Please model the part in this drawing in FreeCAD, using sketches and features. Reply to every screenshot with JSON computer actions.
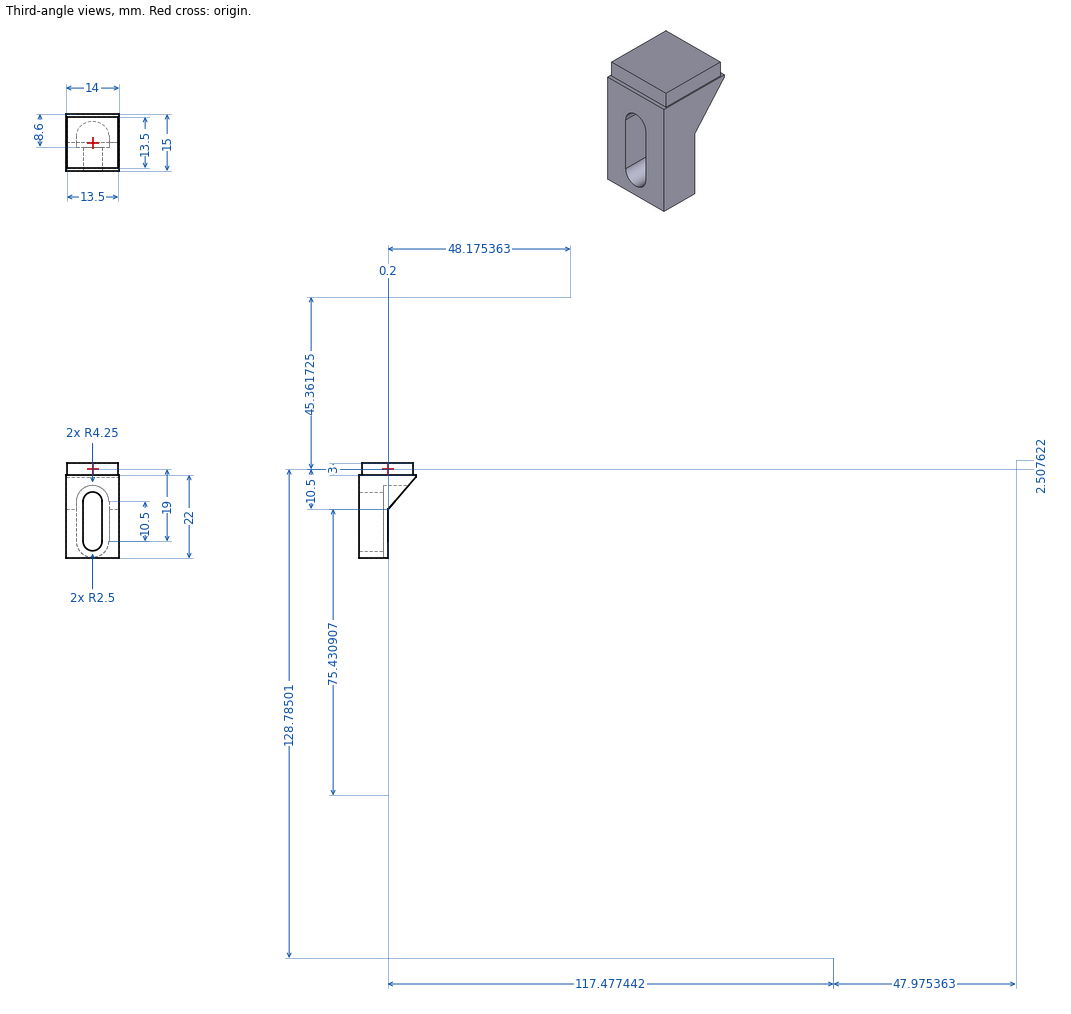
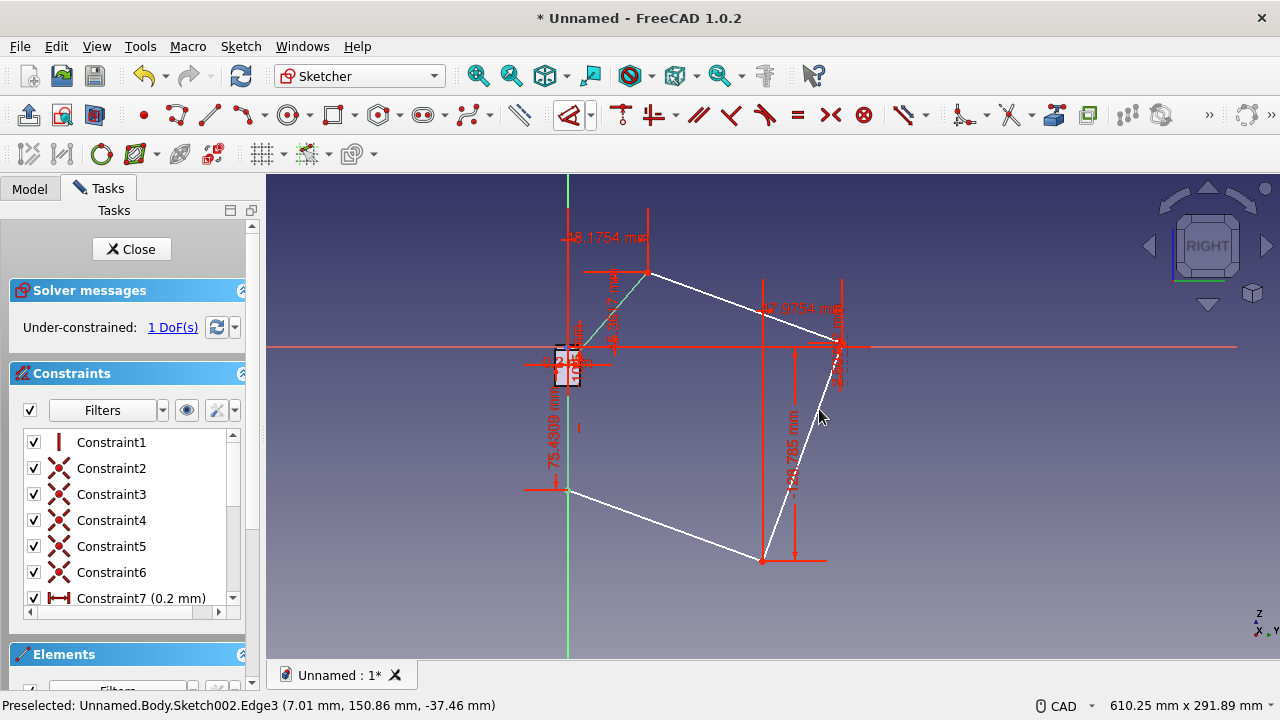
{"action": "left_click", "coordinate": [763, 561]}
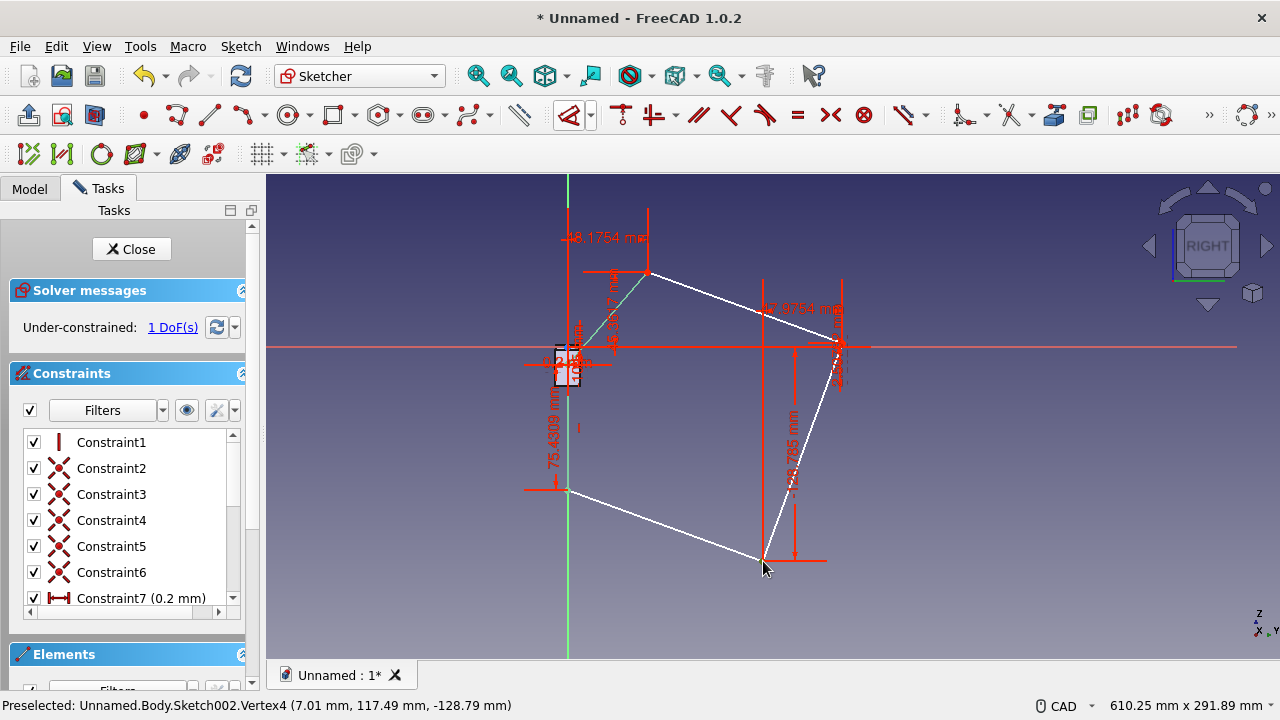
{"action": "key", "text": "l"}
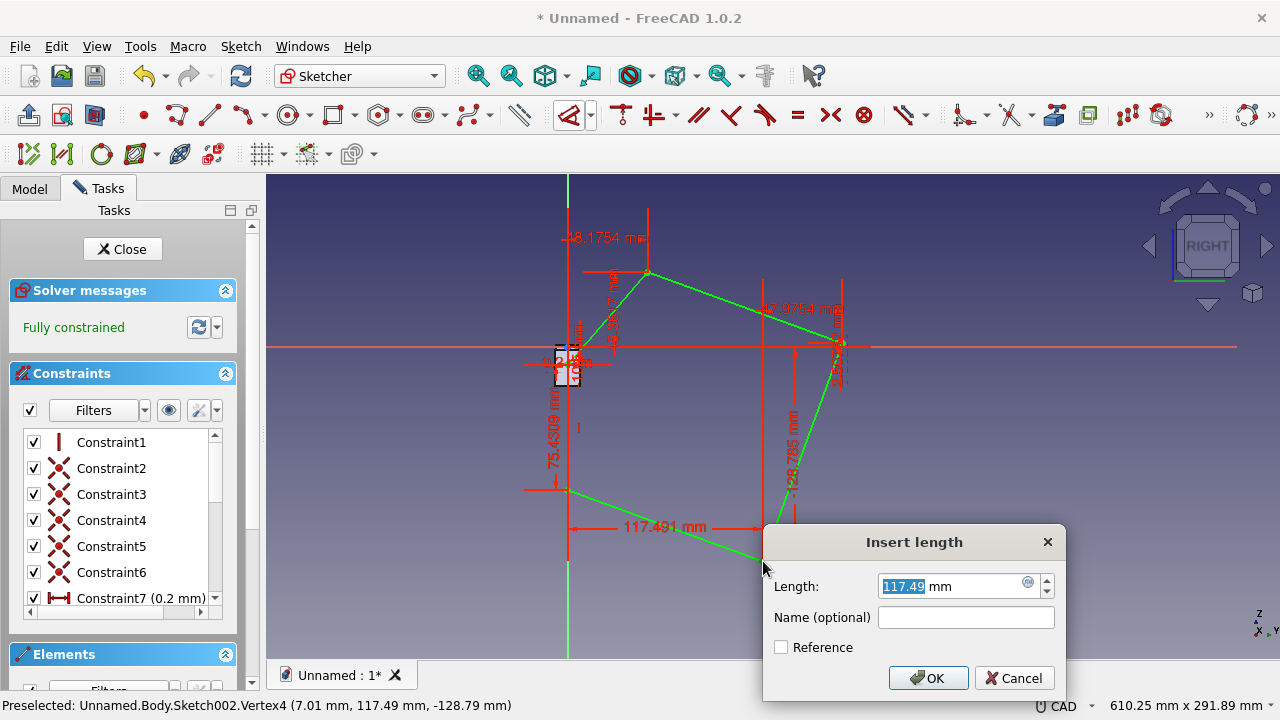
{"action": "type", "text": "117.477442"}
{"action": "key", "text": "Return"}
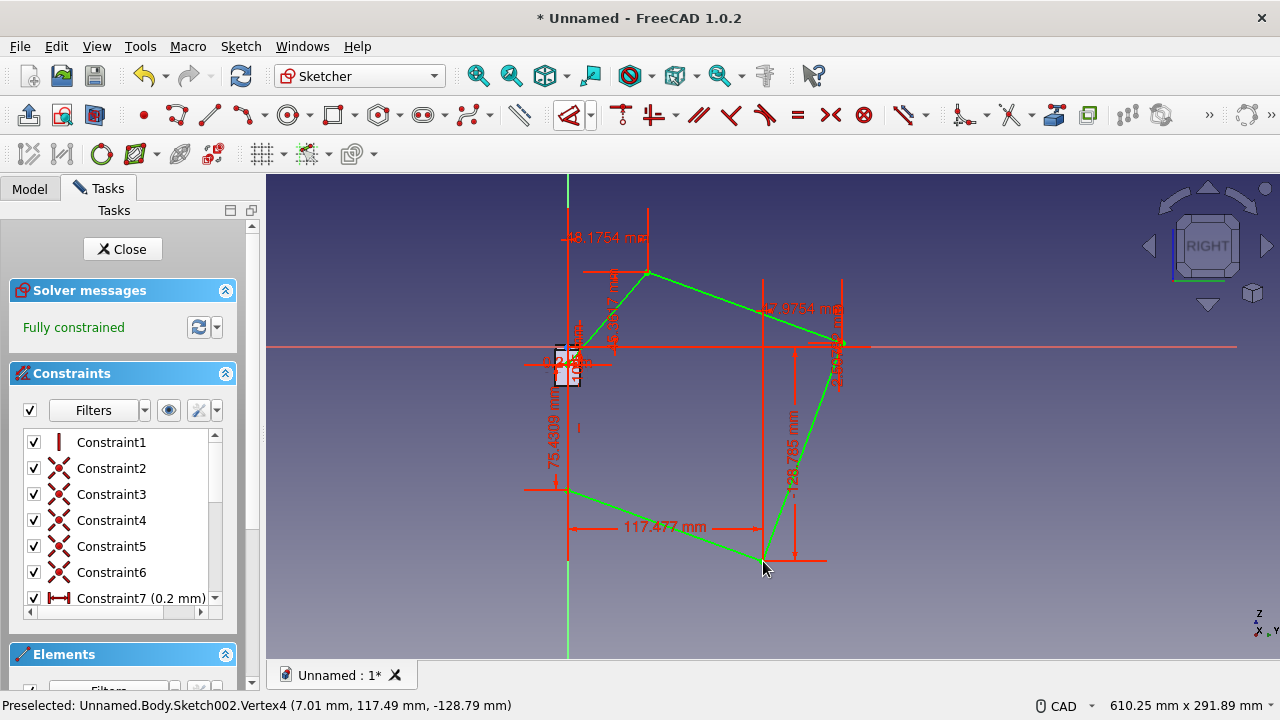
{"action": "left_click", "coordinate": [123, 249]}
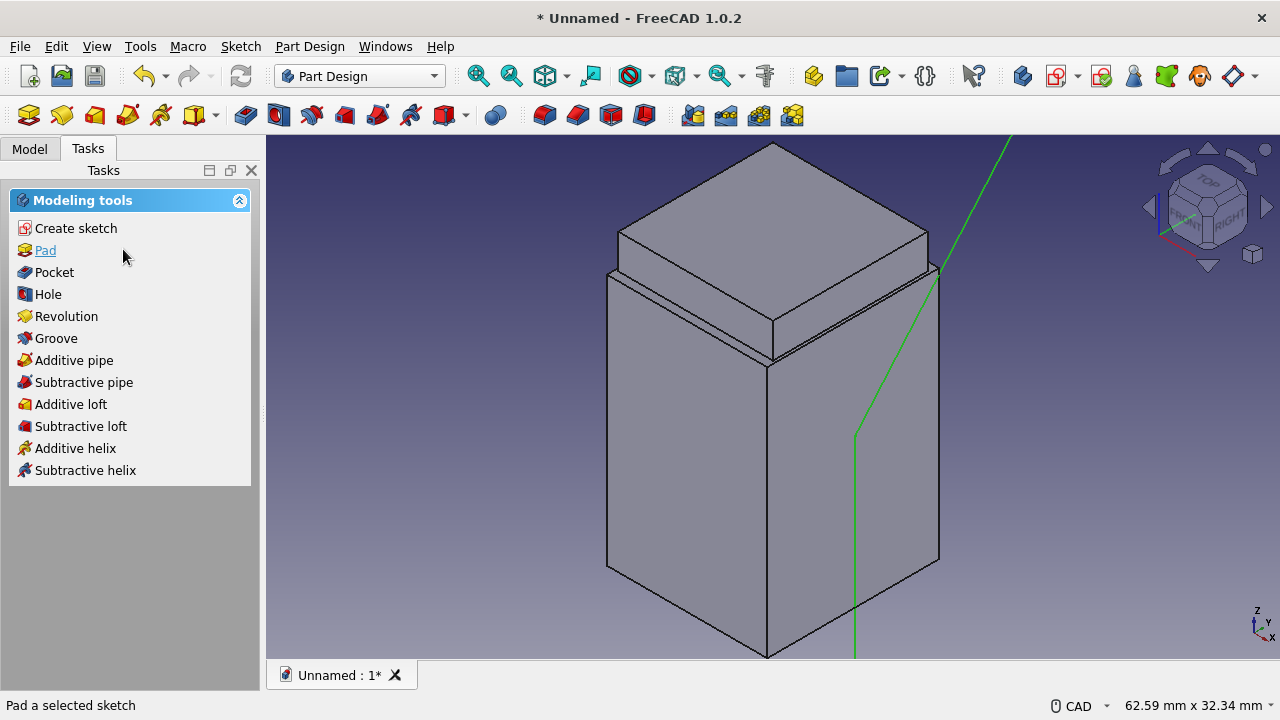
{"action": "left_click", "coordinate": [246, 116]}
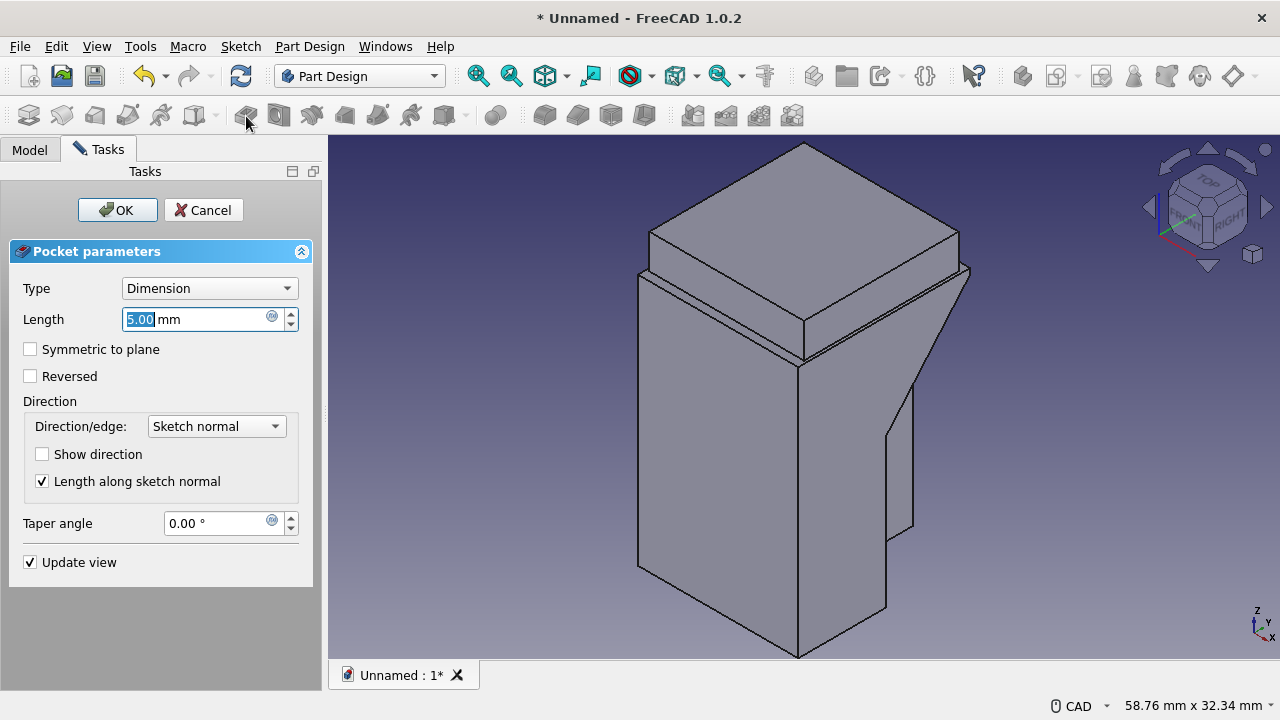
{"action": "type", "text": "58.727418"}
{"action": "key", "text": "Tab"}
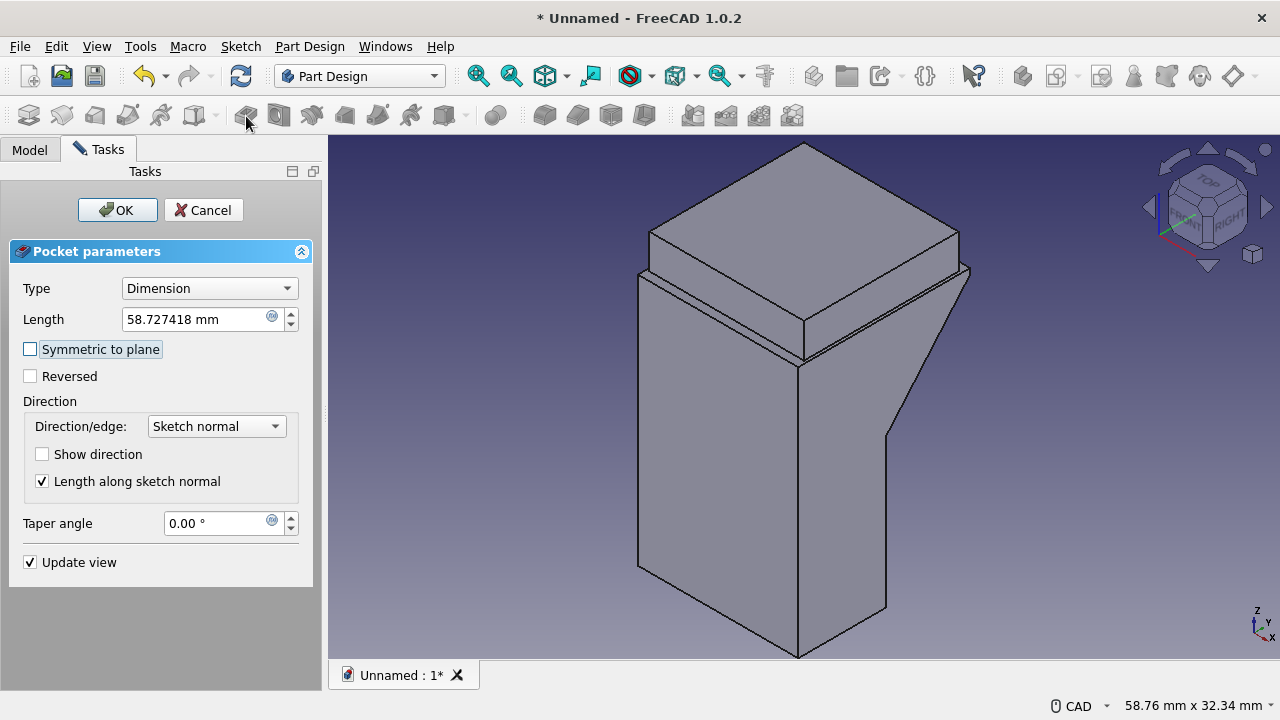
{"action": "left_click", "coordinate": [31, 349]}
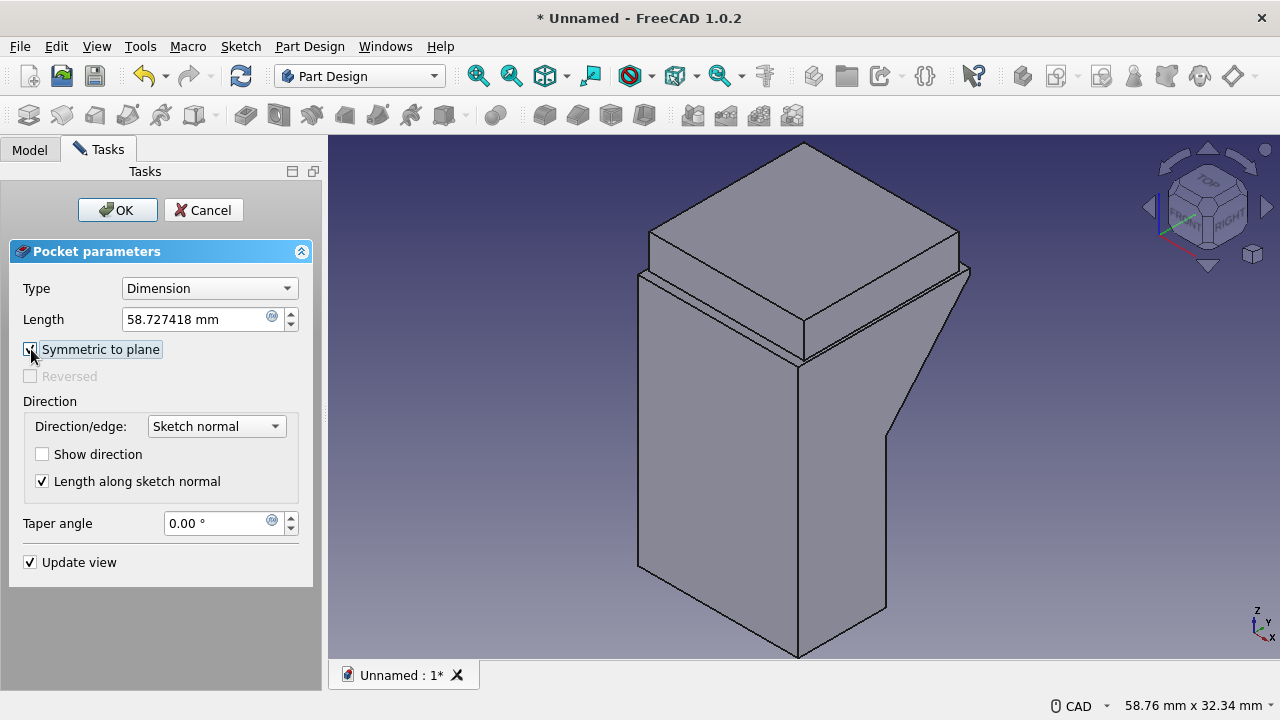
{"action": "left_click", "coordinate": [118, 210]}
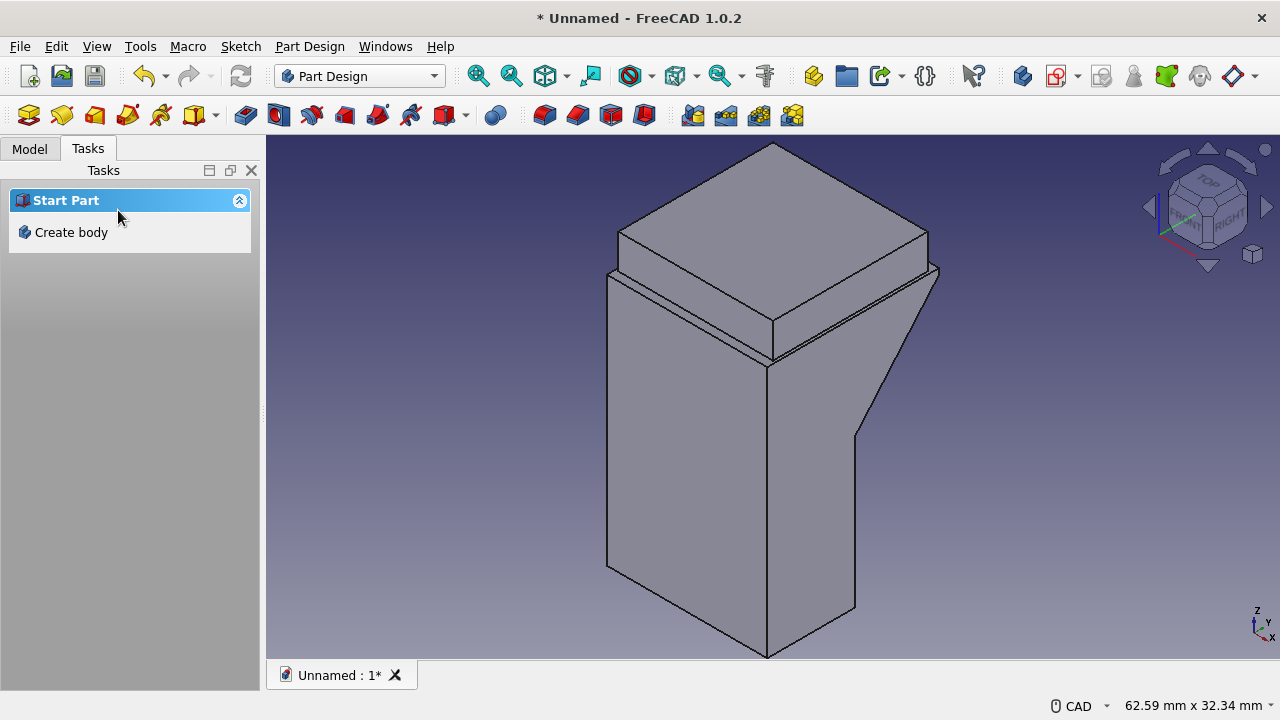
{"action": "key", "text": "4"}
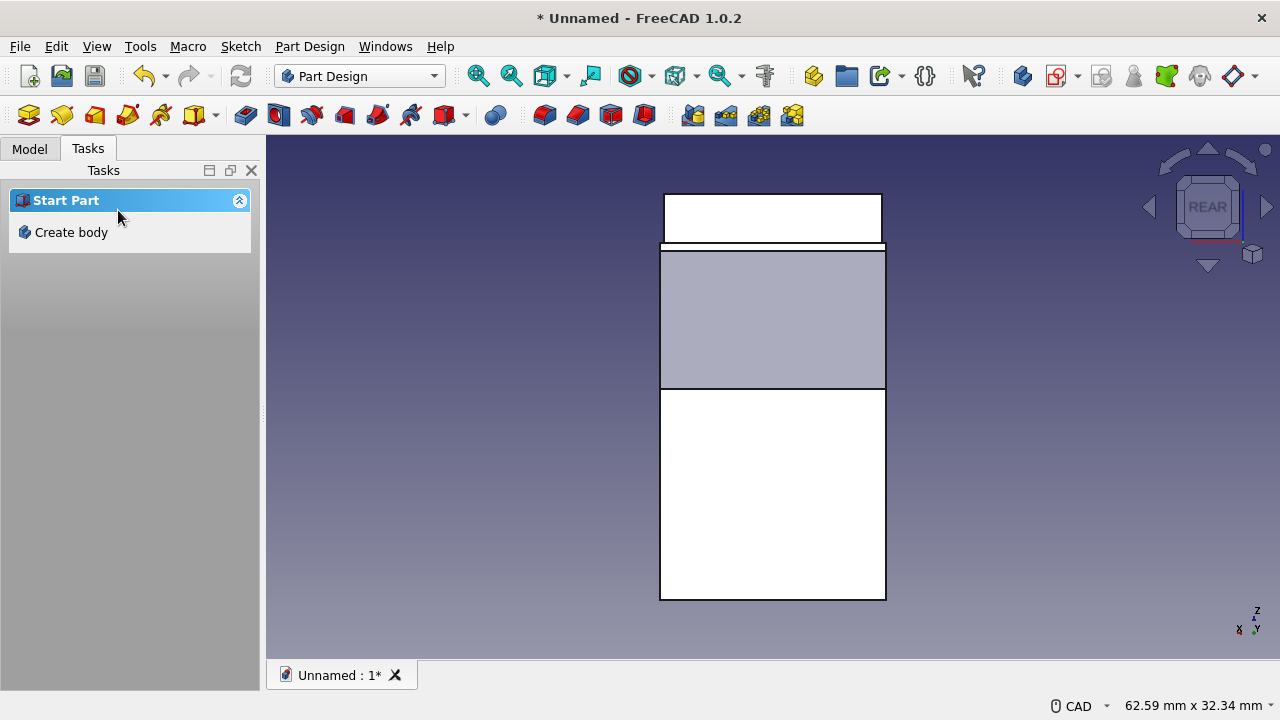
{"action": "scroll", "coordinate": [676, 246], "scroll_direction": "up", "scroll_amount": 6}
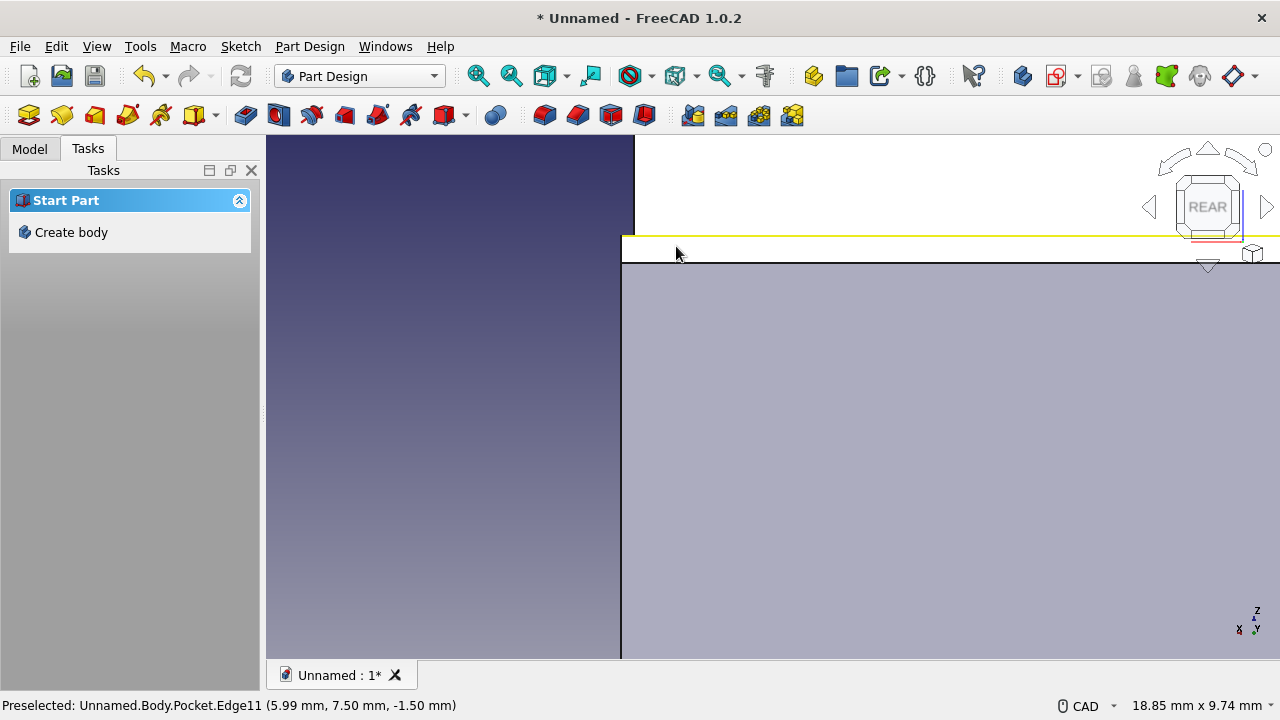
{"action": "left_click", "coordinate": [674, 248]}